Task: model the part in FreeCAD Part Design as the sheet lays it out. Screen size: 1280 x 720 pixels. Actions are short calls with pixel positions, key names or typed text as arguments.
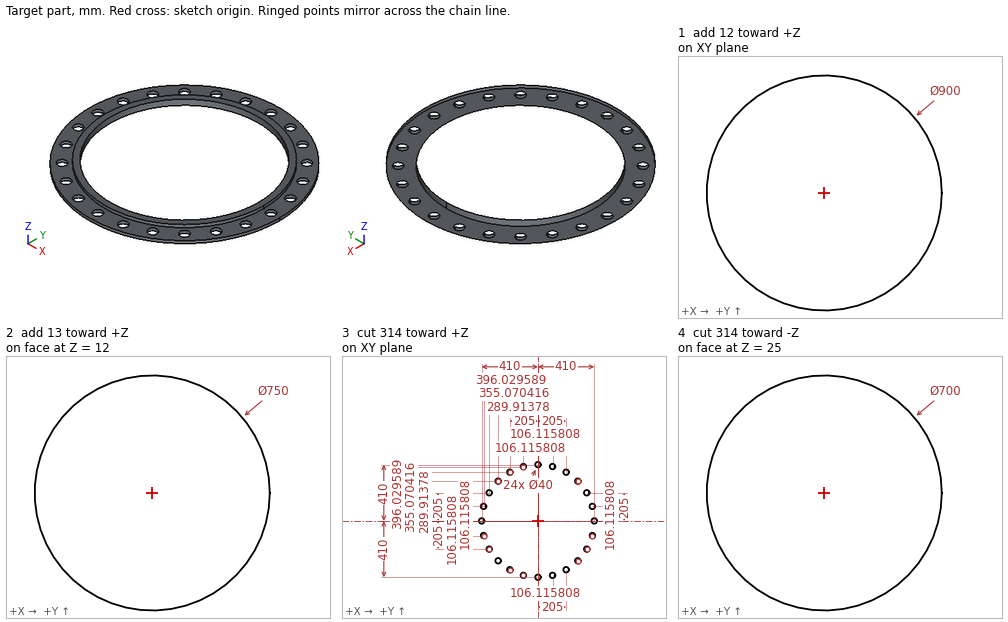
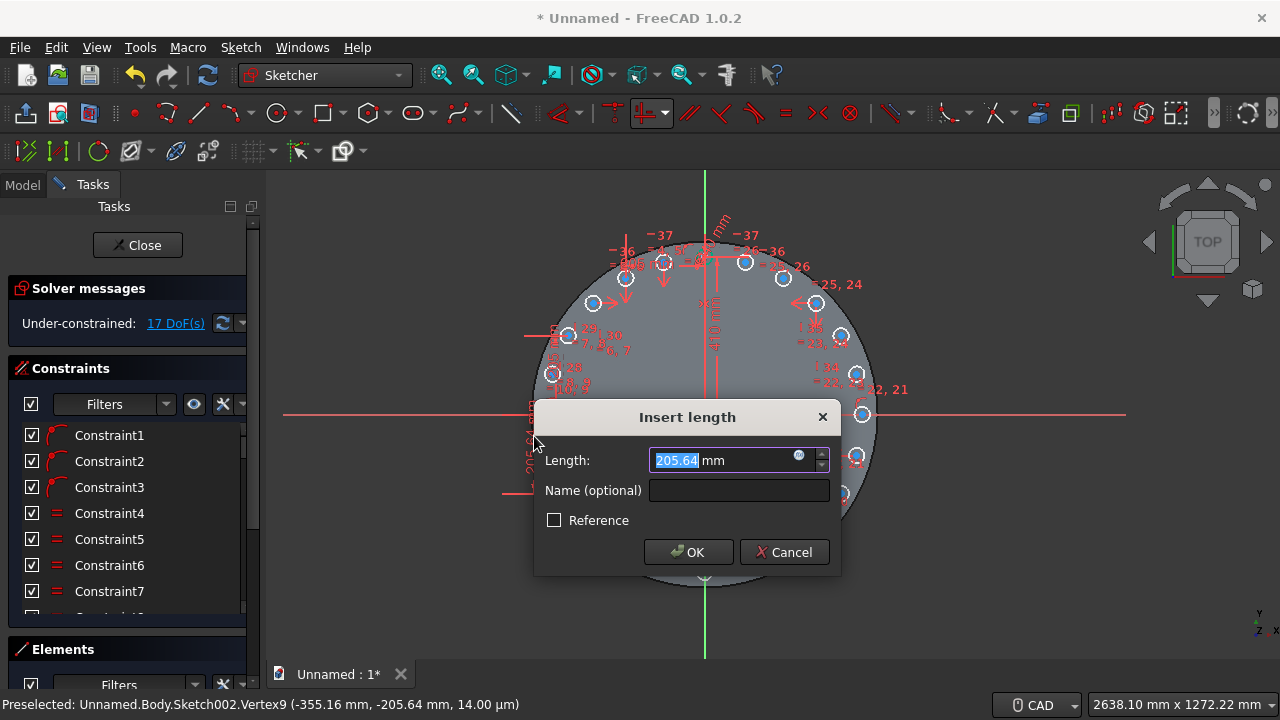
text(205)
key(Return)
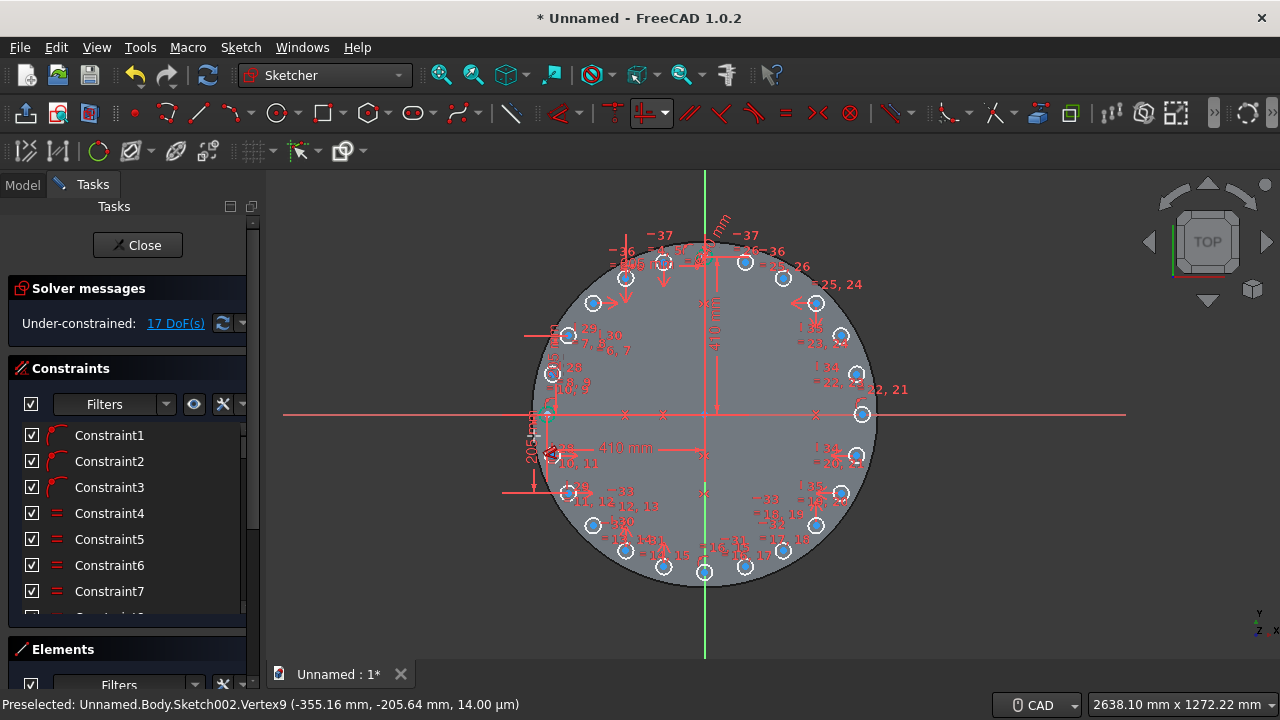
click(705, 572)
click(739, 494)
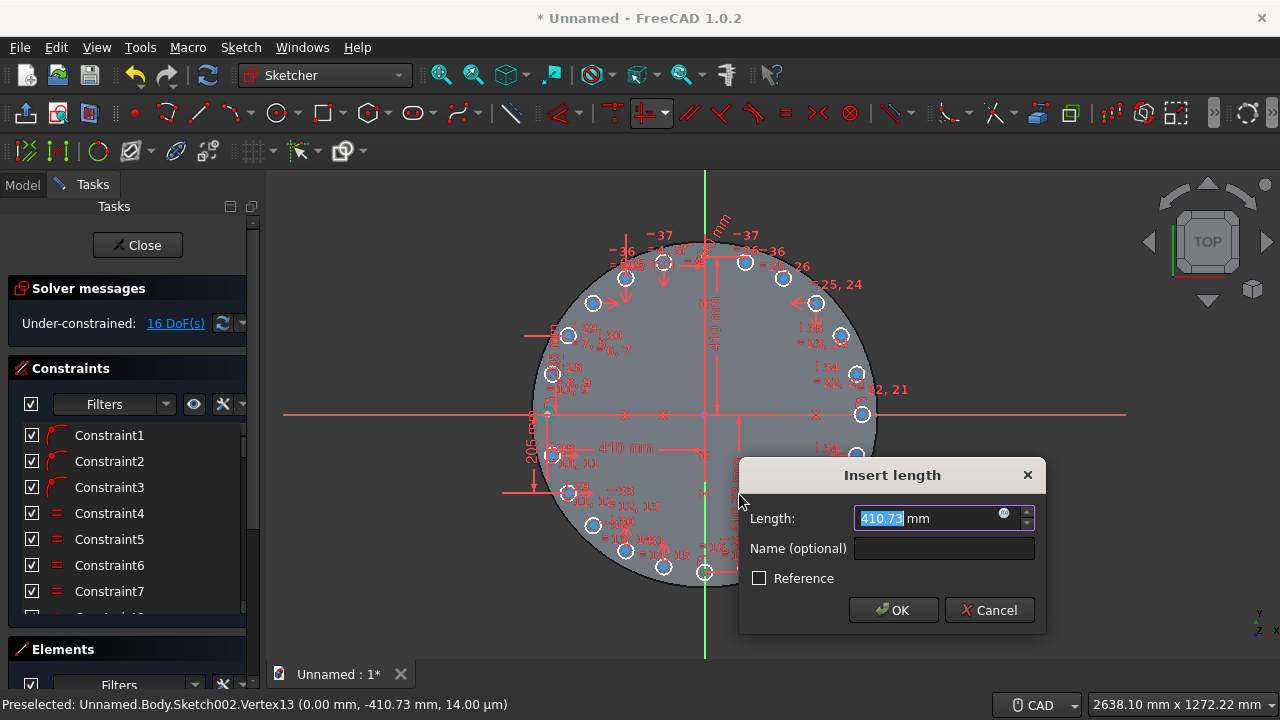
text(410)
key(Return)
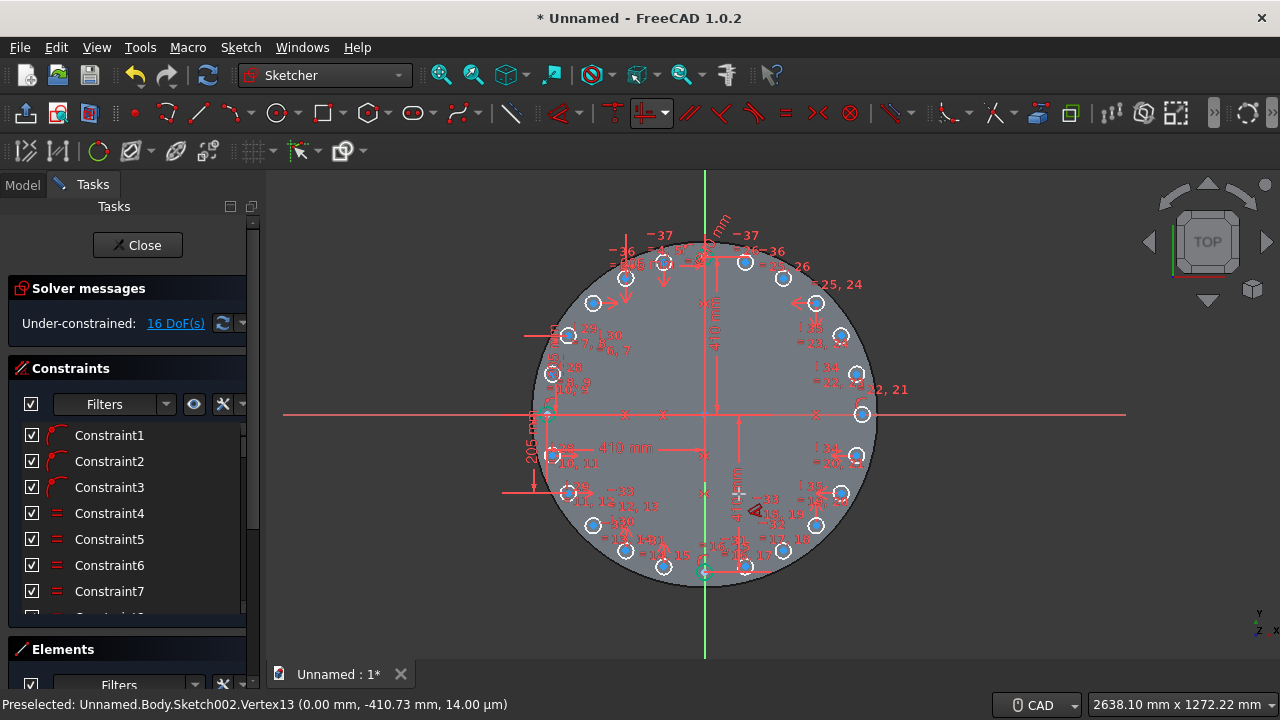
click(783, 551)
click(726, 585)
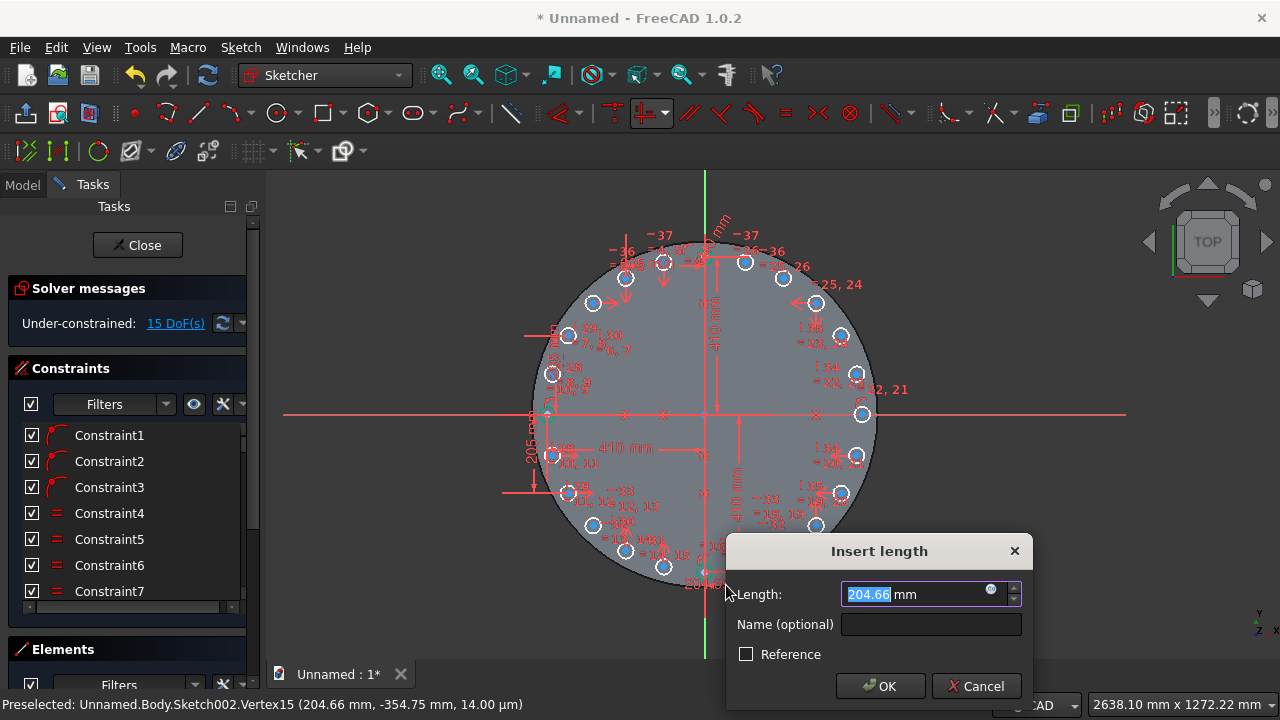
text(205)
key(Return)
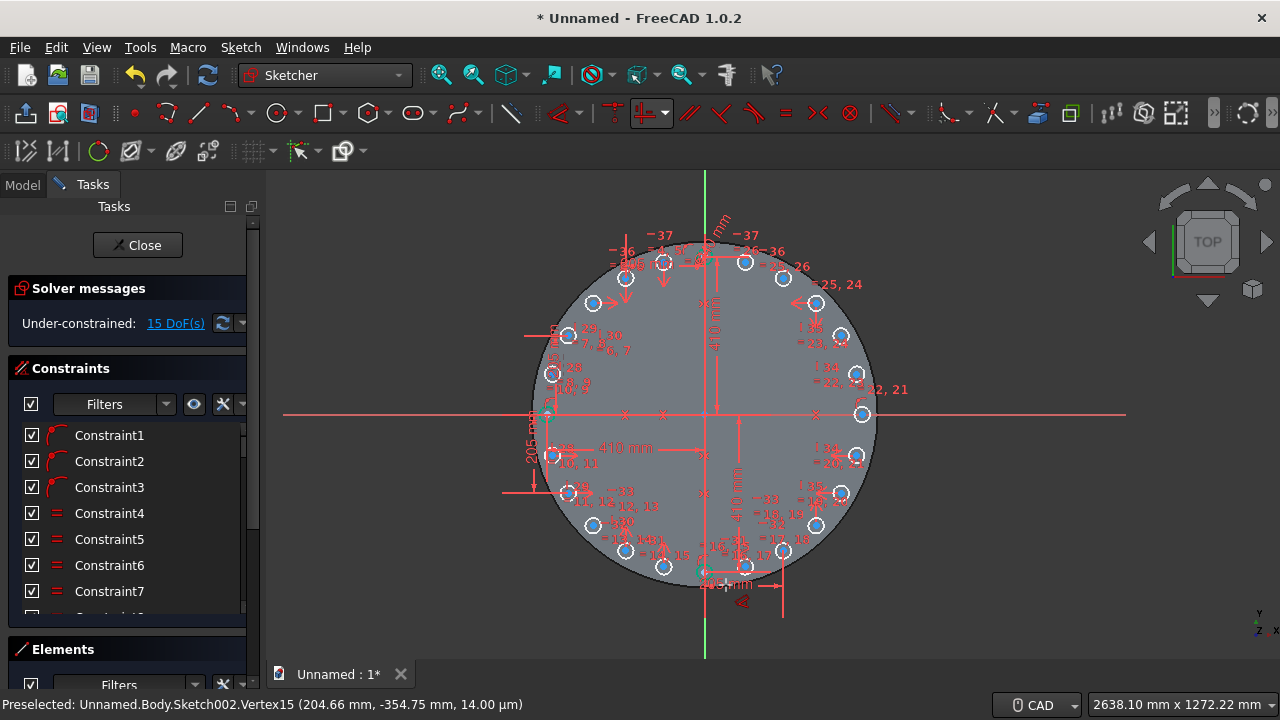
click(862, 415)
click(783, 449)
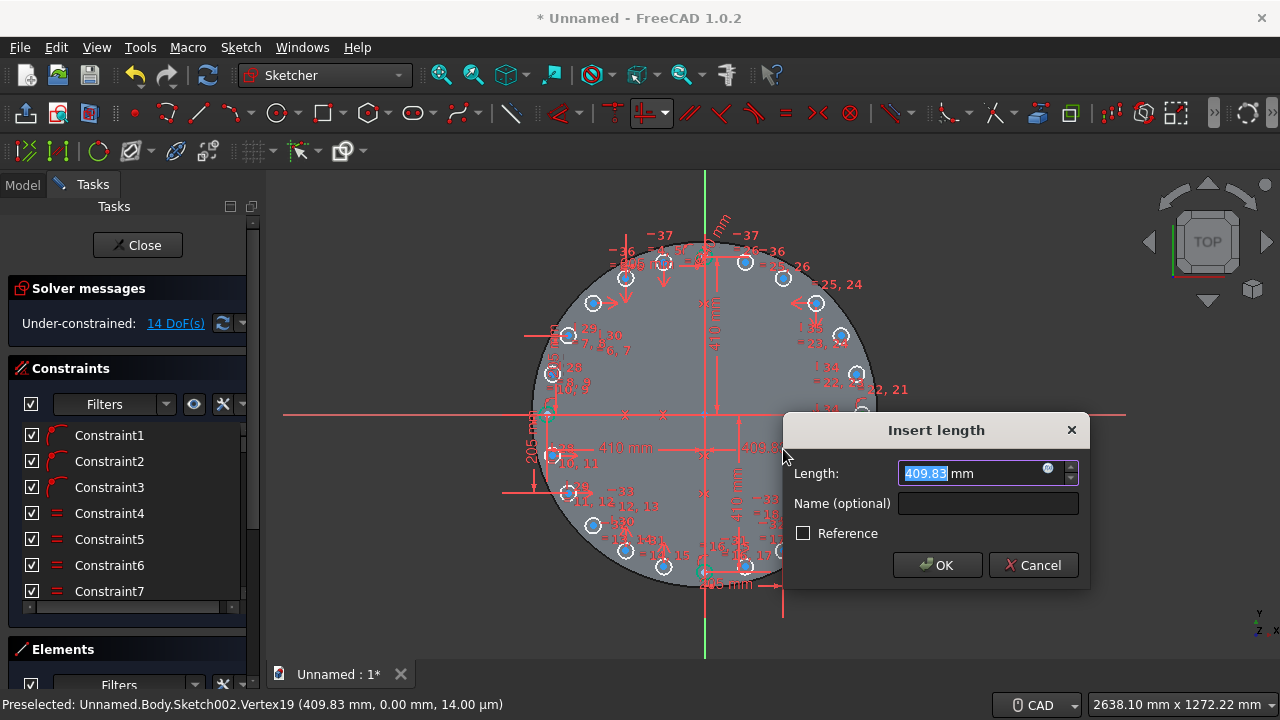
text(410)
key(Return)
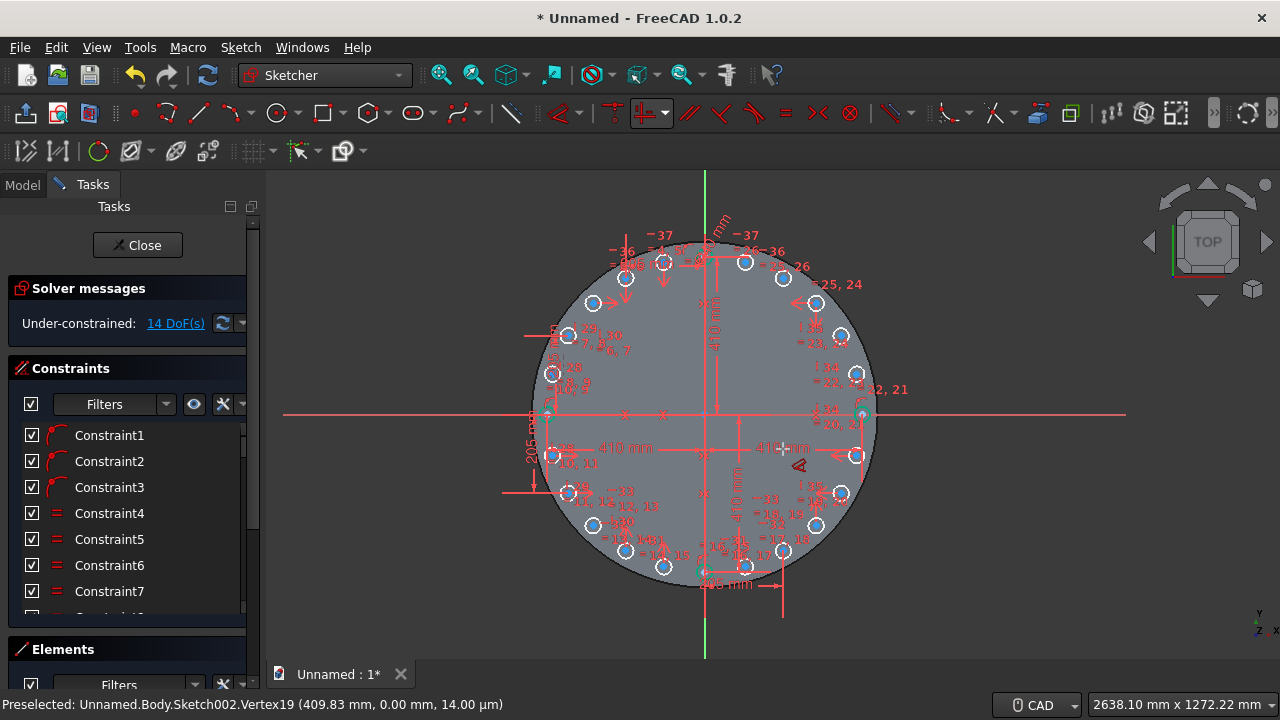
click(841, 336)
click(875, 357)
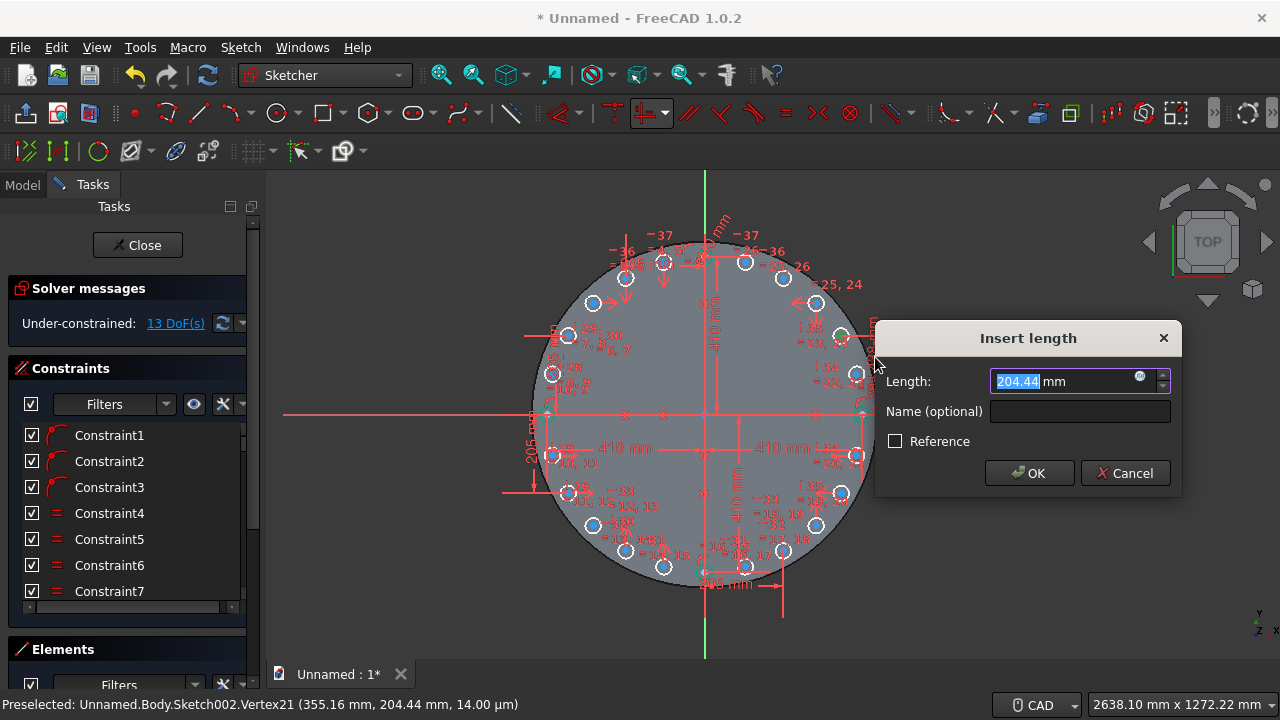
text(205)
key(Return)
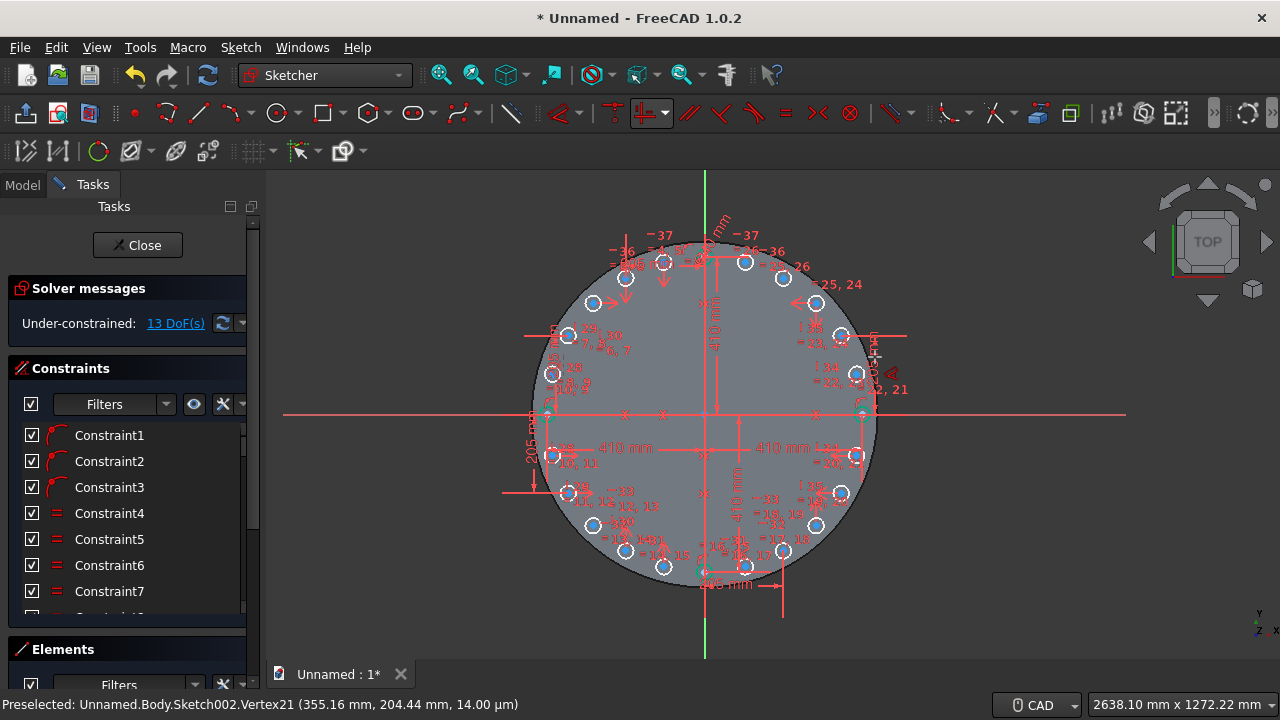
click(783, 278)
click(744, 220)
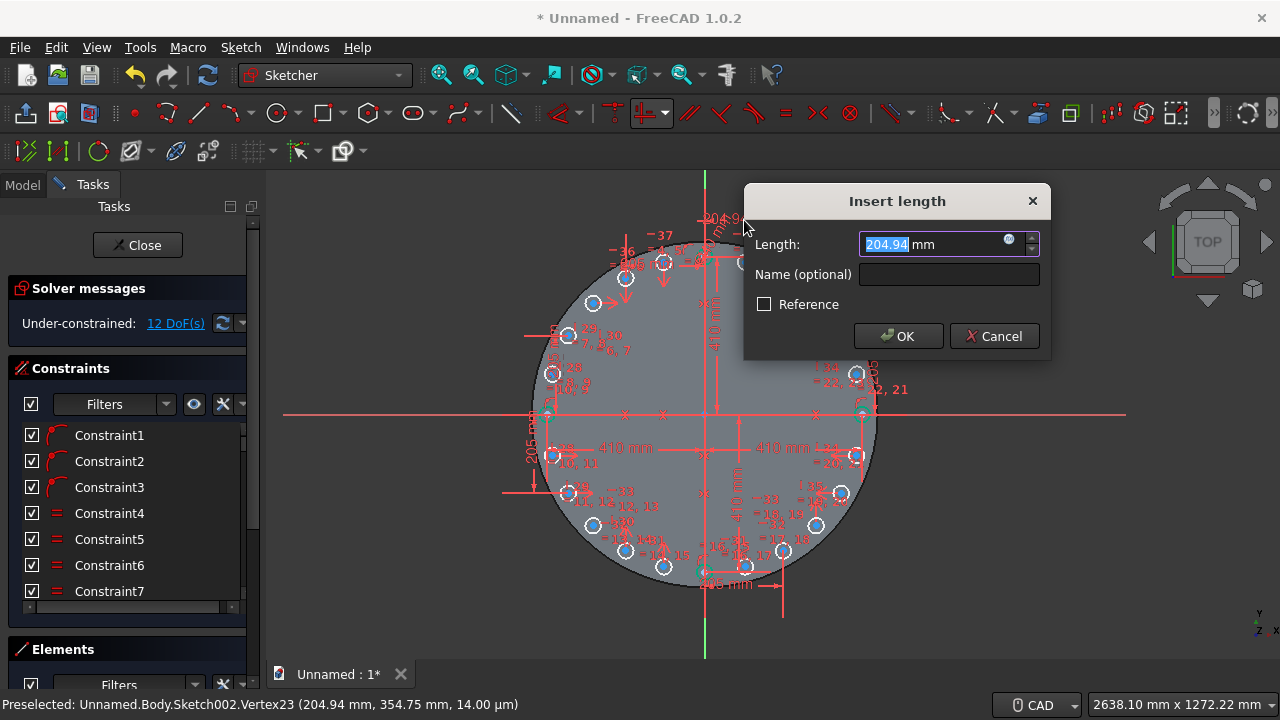
text(205)
key(Return)